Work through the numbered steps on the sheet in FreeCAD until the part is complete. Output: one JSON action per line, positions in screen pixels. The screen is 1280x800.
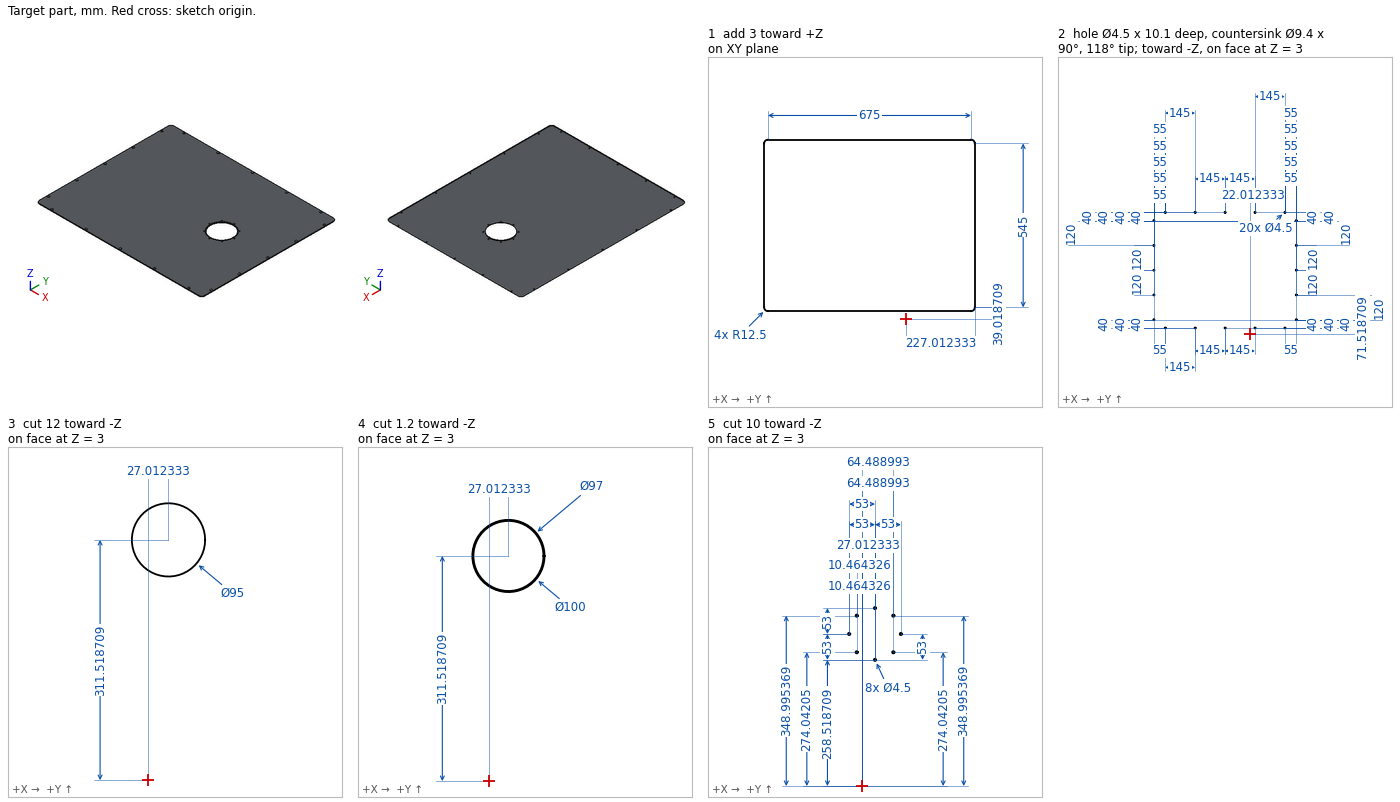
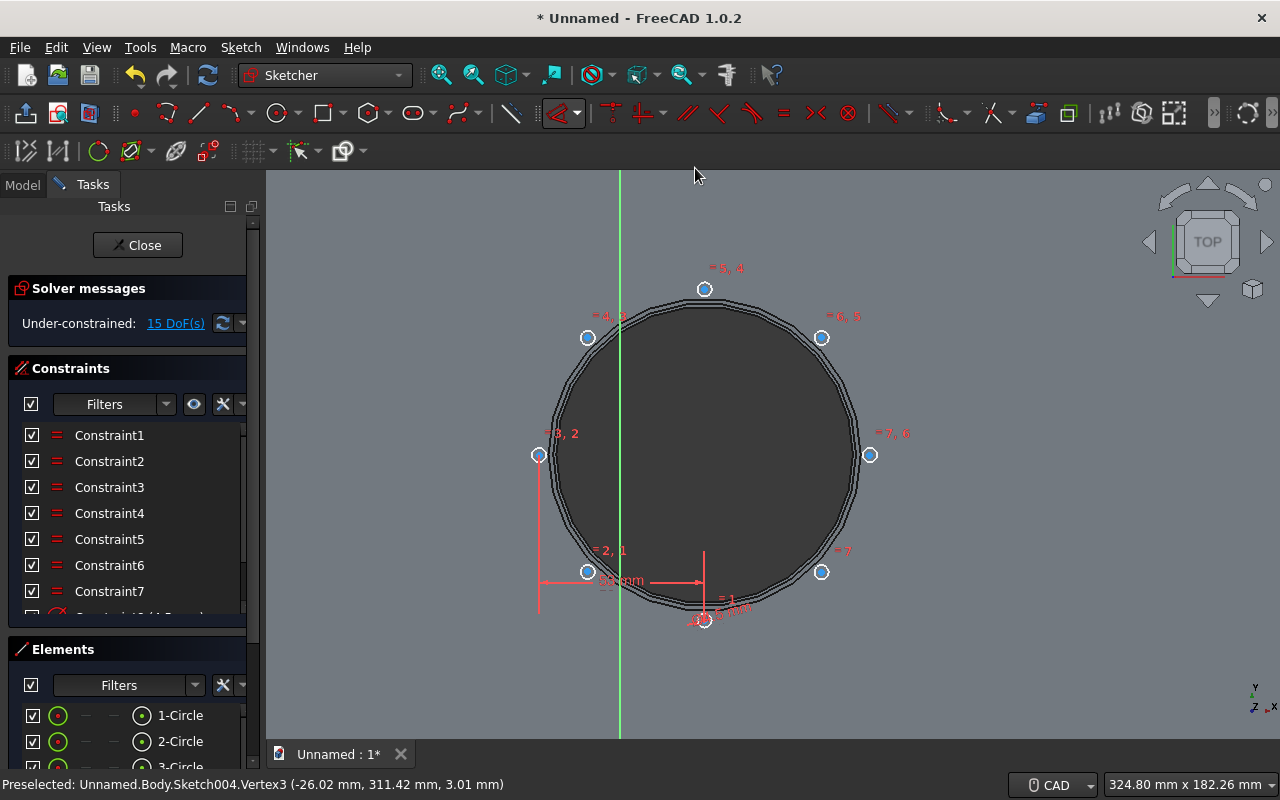
{"action": "left_click", "coordinate": [704, 620]}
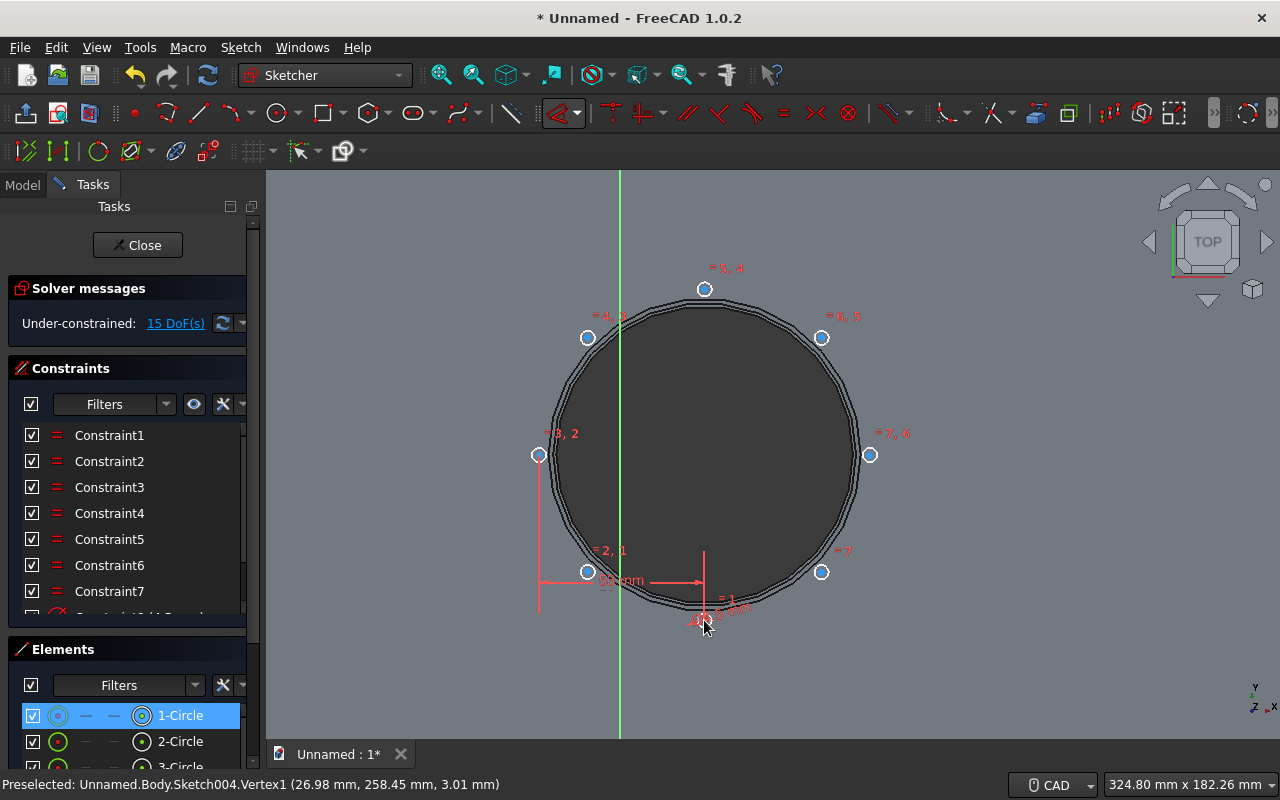
{"action": "left_click", "coordinate": [539, 455]}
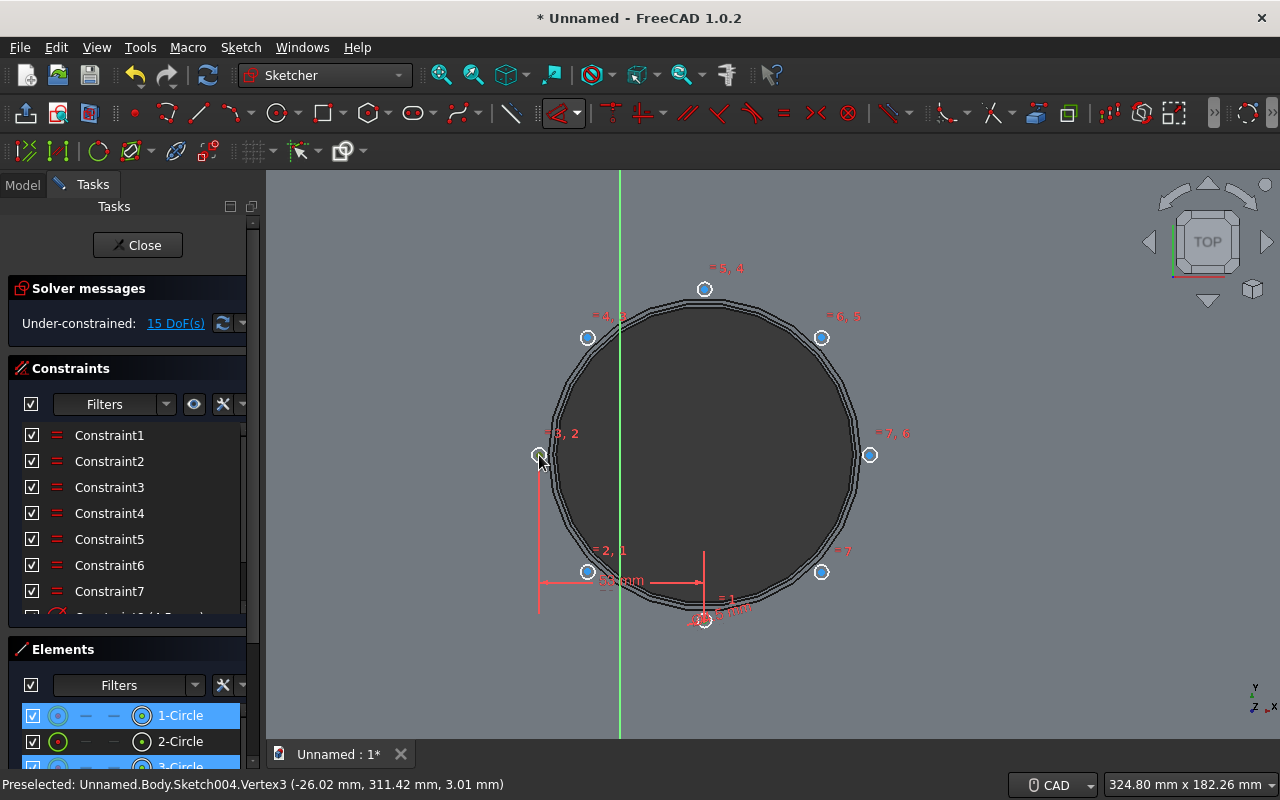
{"action": "key", "text": "i"}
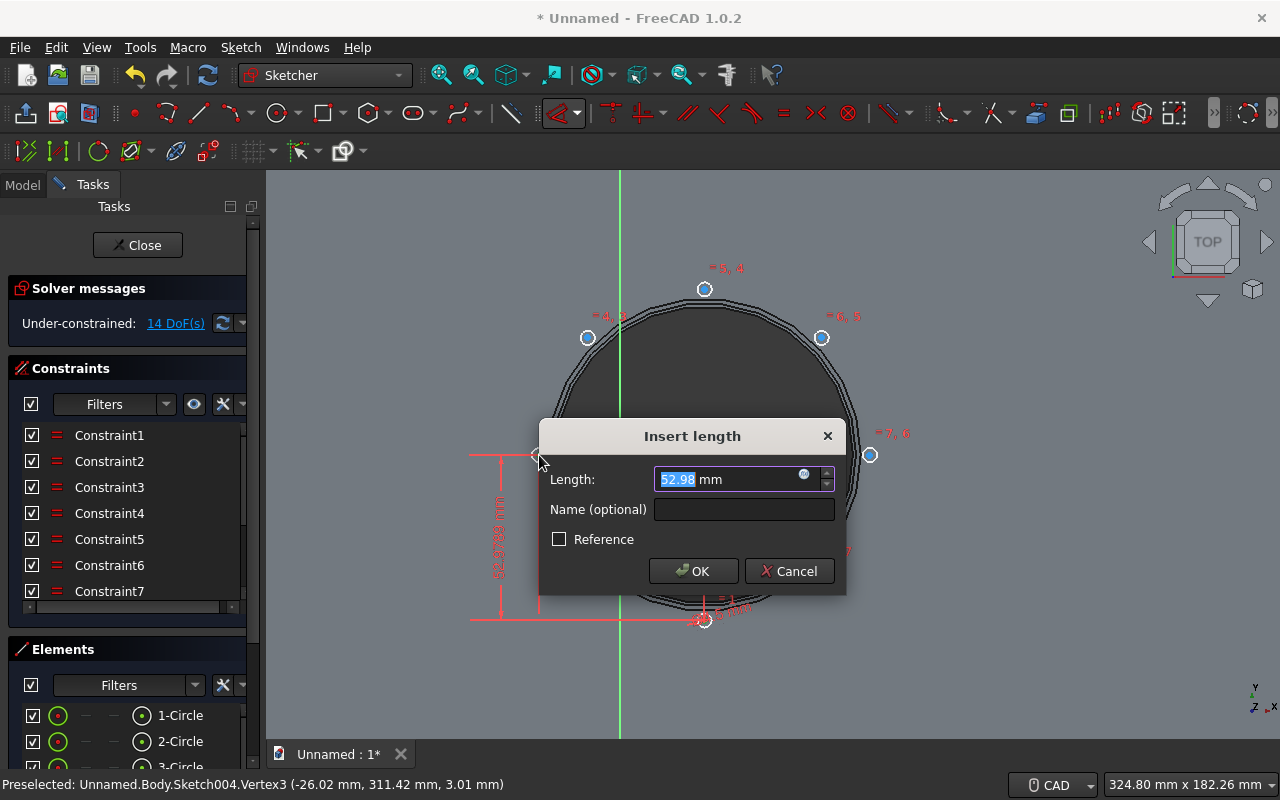
{"action": "type", "text": "53"}
{"action": "key", "text": "Return"}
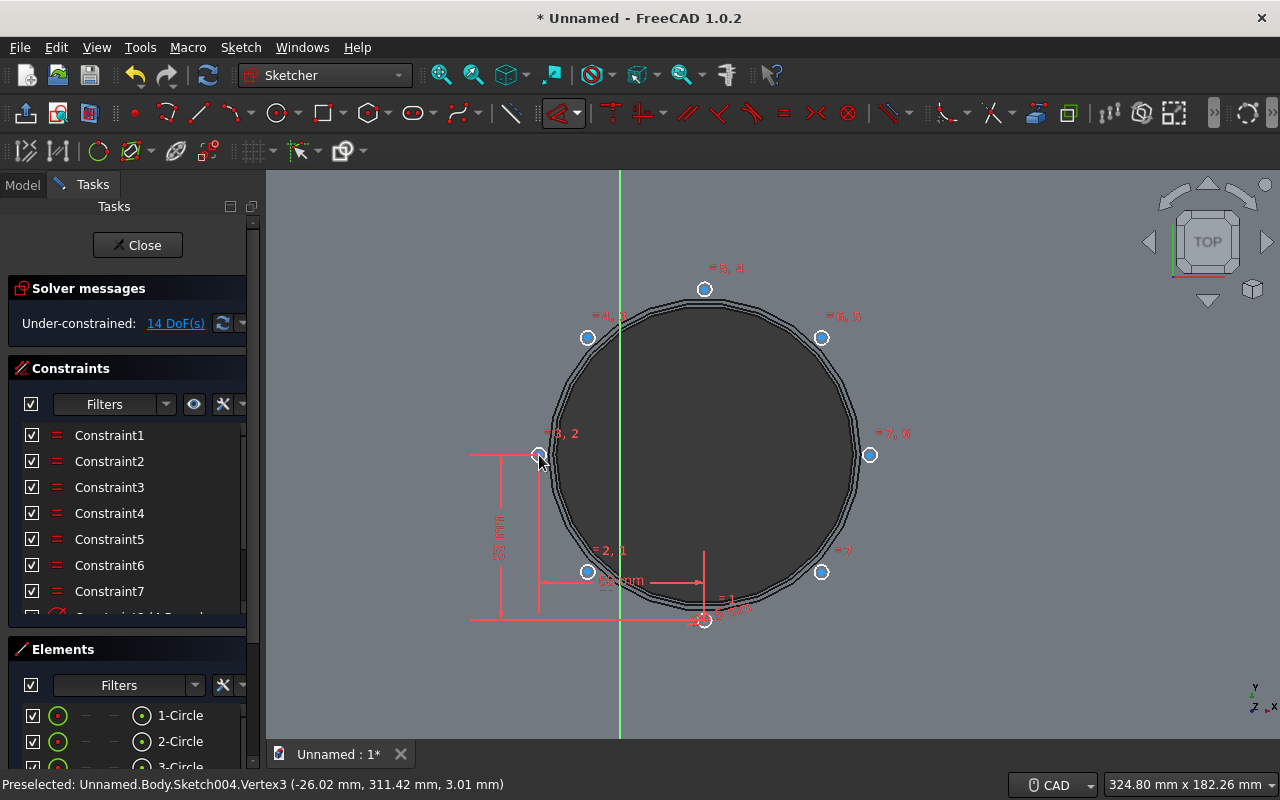
{"action": "left_click", "coordinate": [539, 455]}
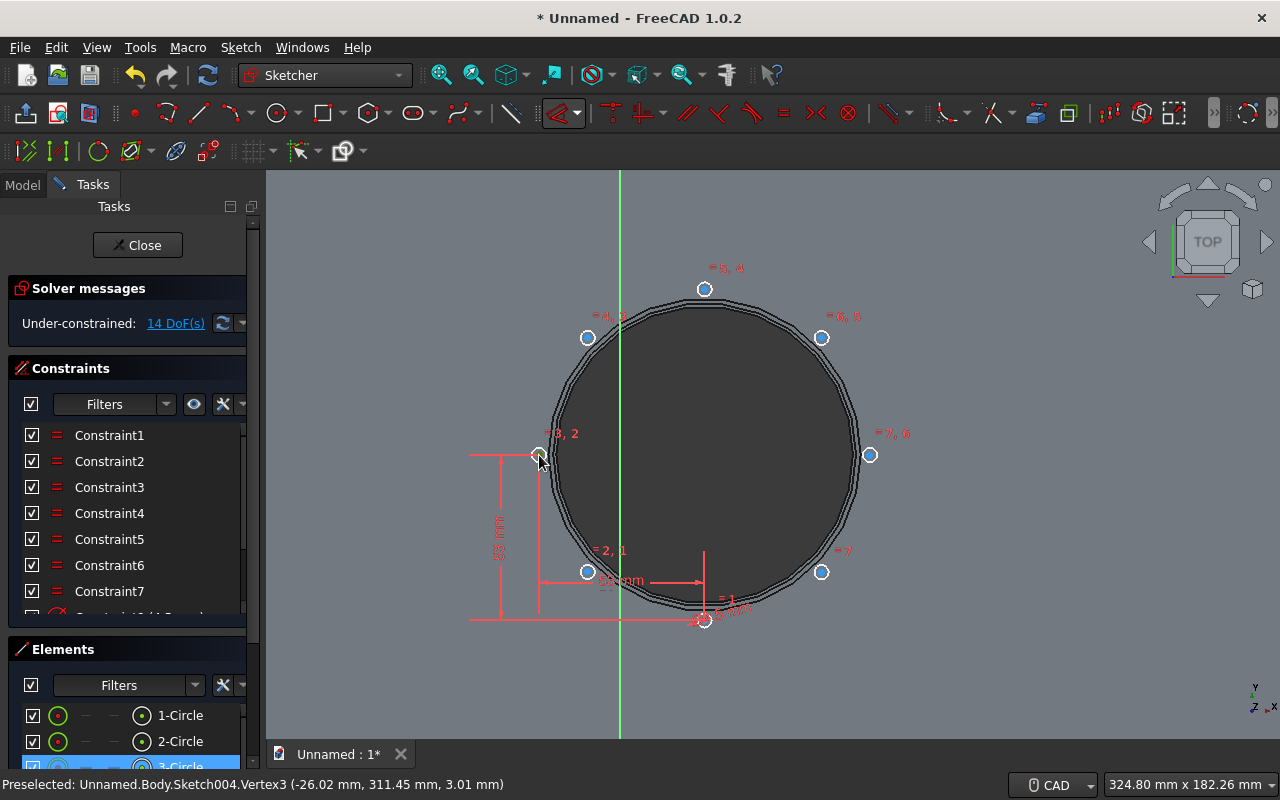
{"action": "left_click", "coordinate": [705, 289]}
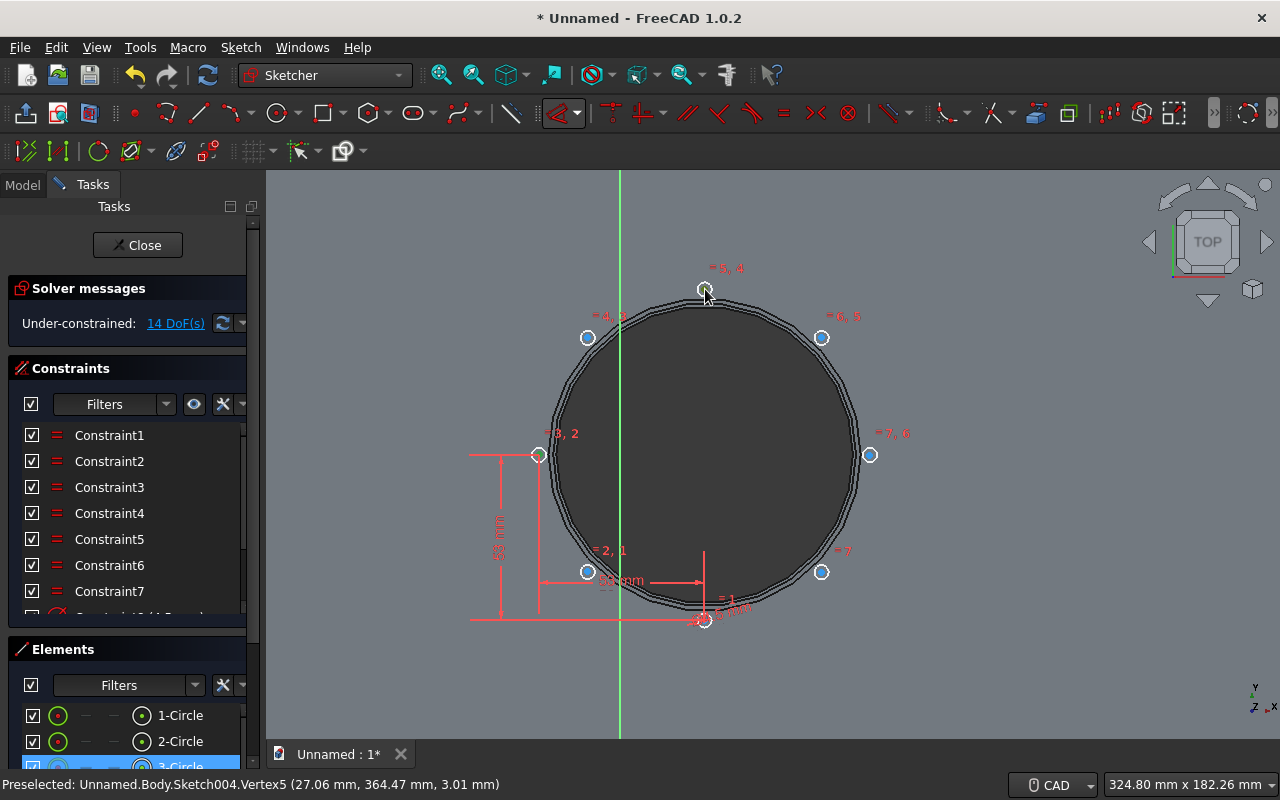
{"action": "key", "text": "l"}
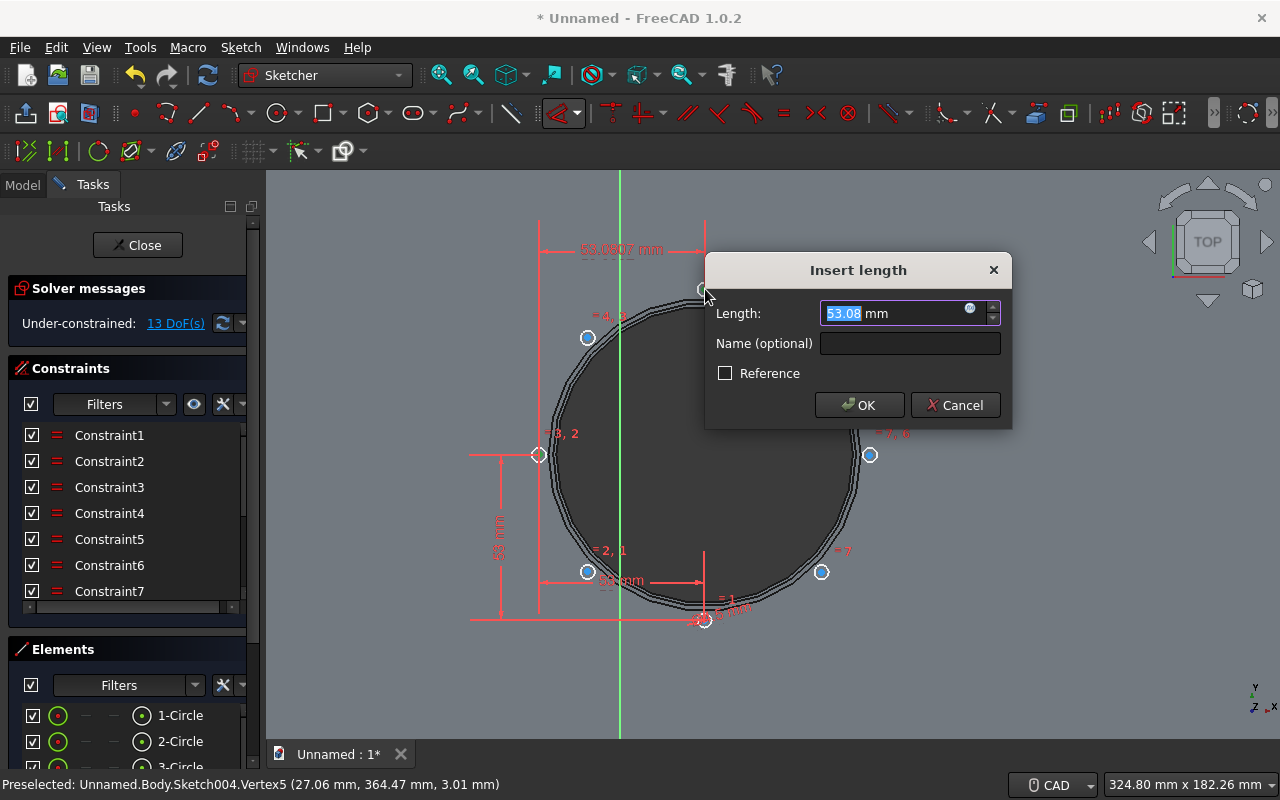
{"action": "type", "text": "53"}
{"action": "key", "text": "Return"}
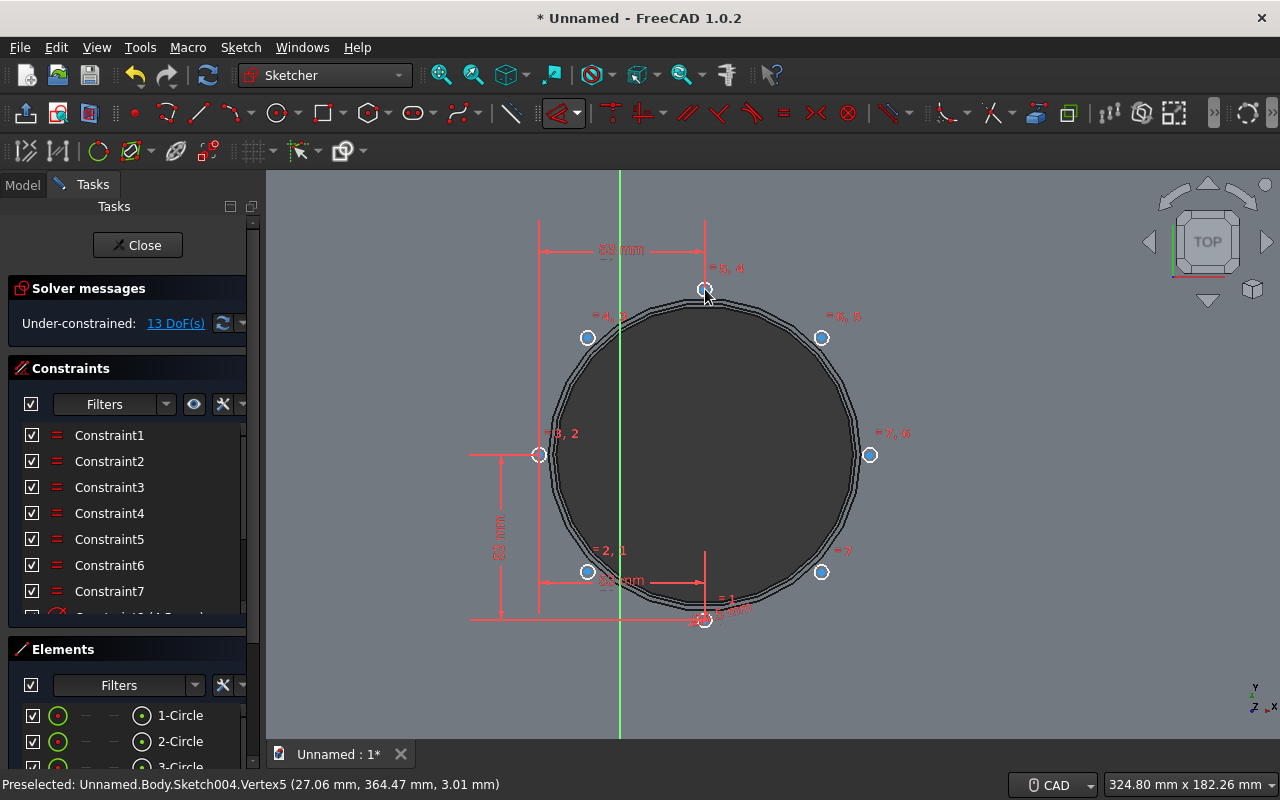
{"action": "left_click", "coordinate": [539, 455]}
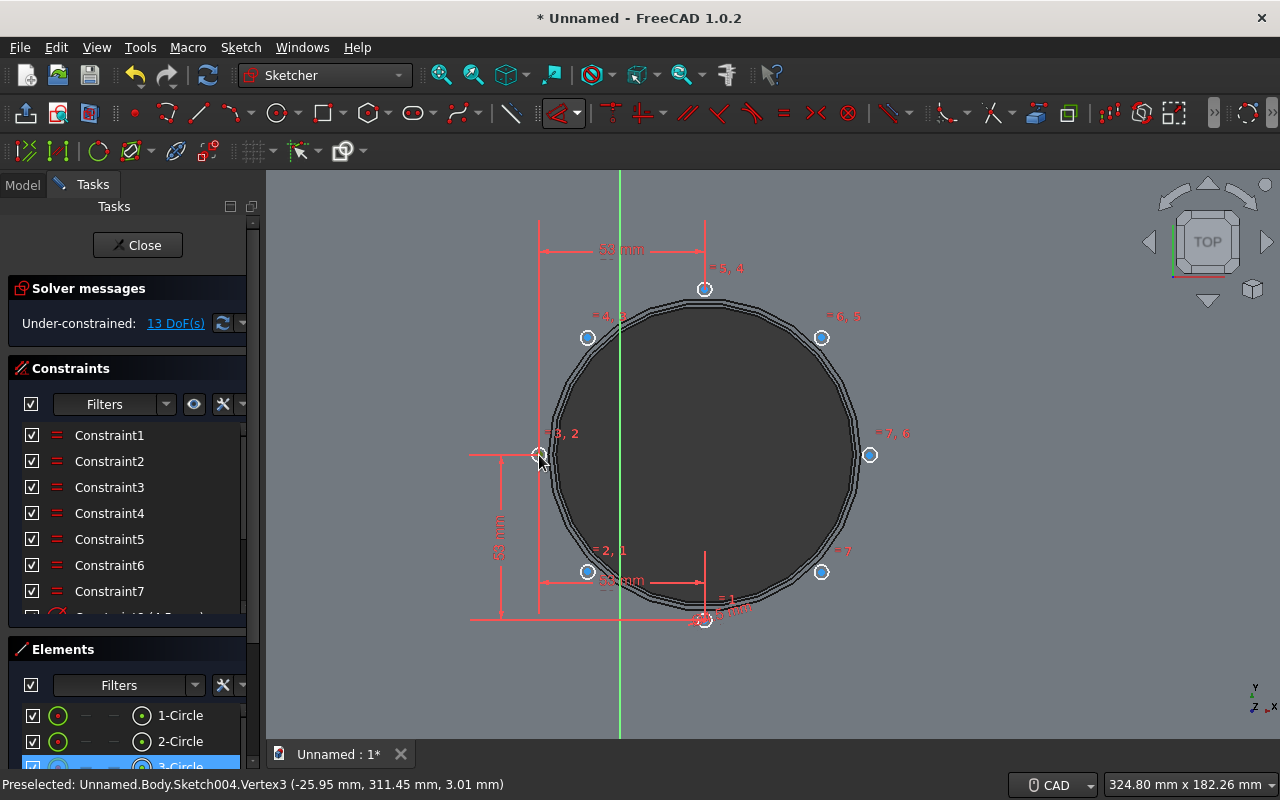
{"action": "left_click", "coordinate": [705, 289]}